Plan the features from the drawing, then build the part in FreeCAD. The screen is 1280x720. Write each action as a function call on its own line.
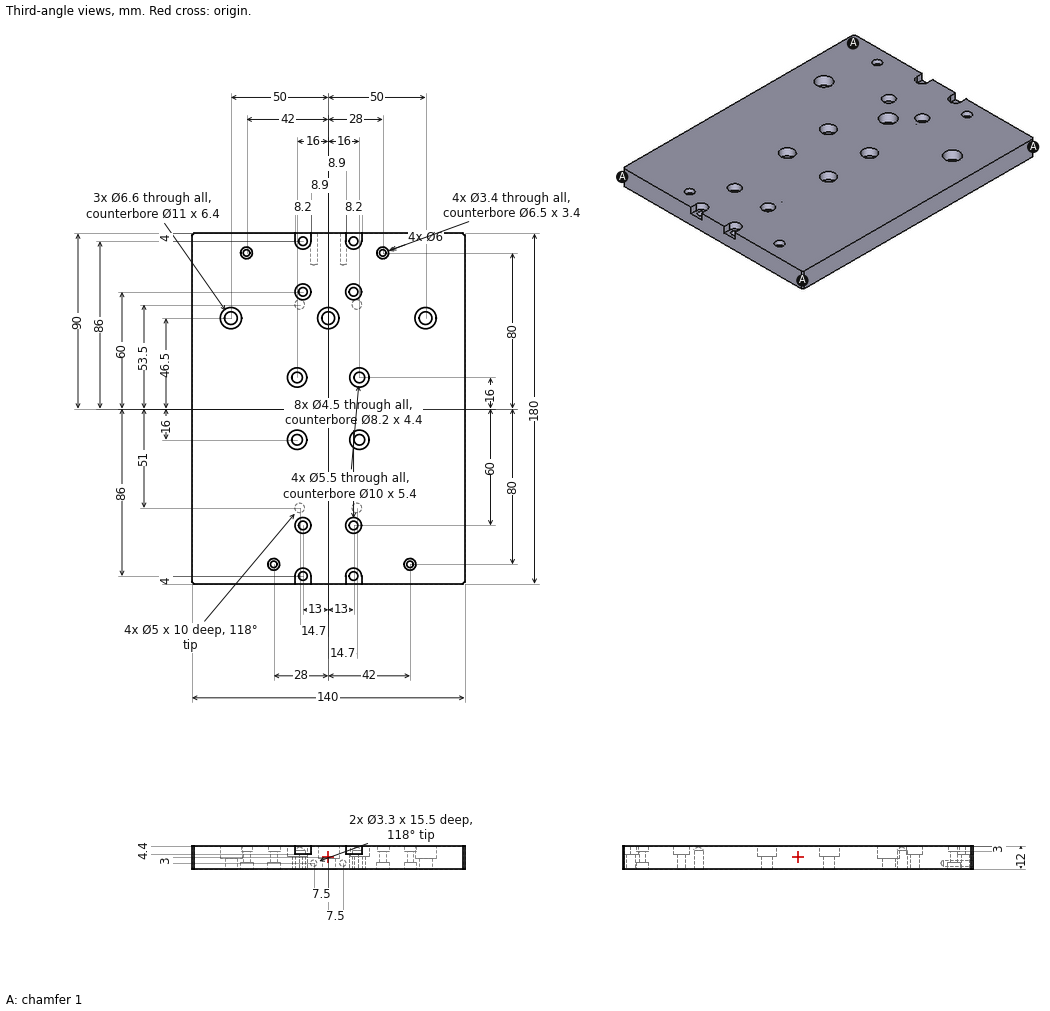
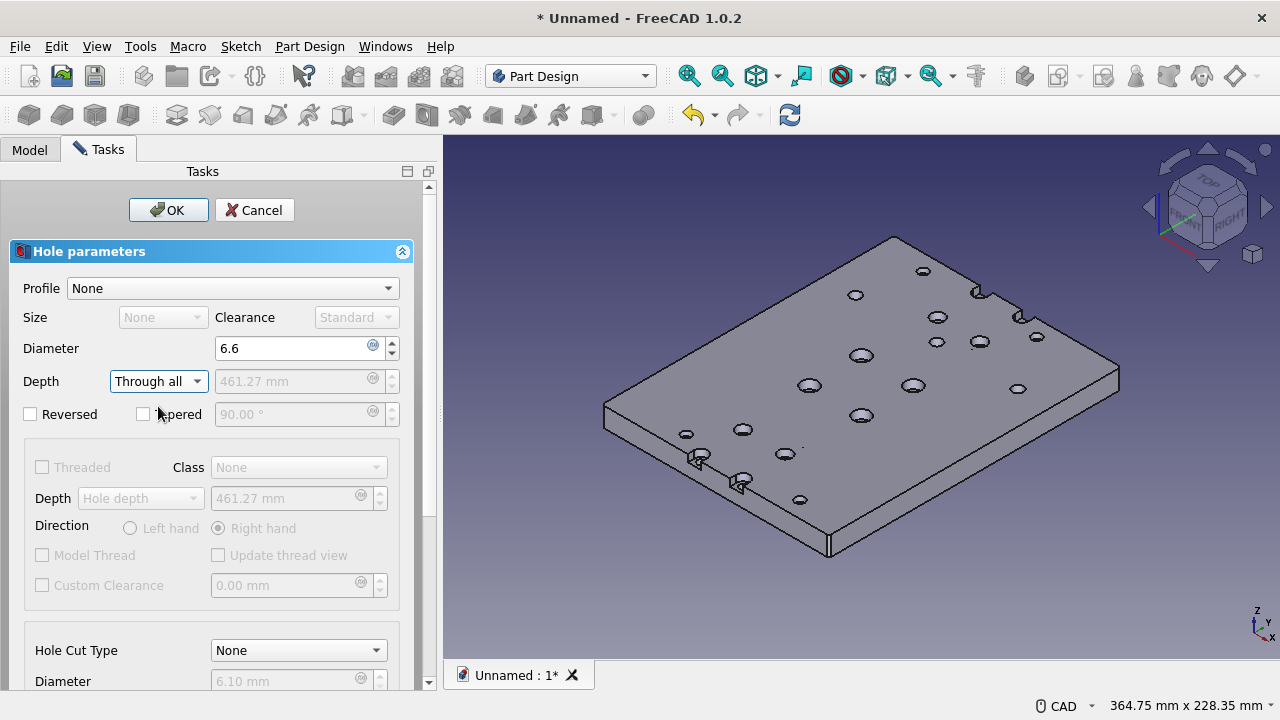
click(300, 650)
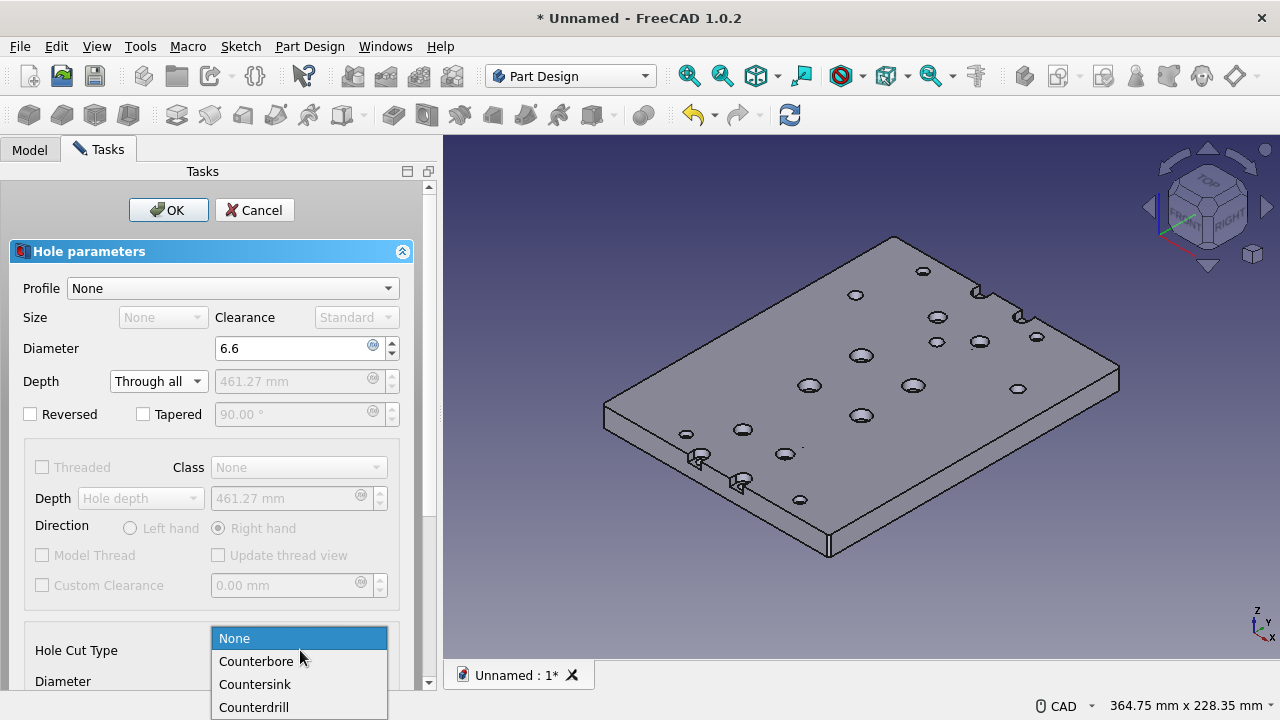
click(298, 662)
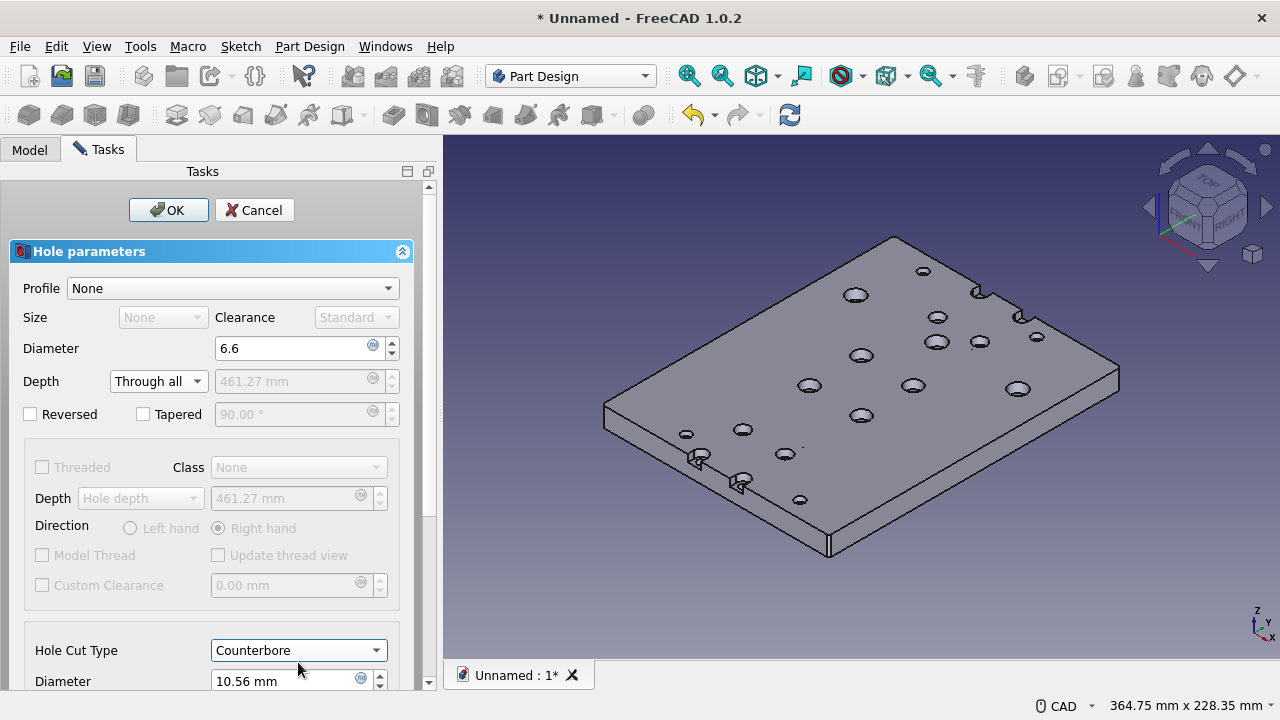
scroll(429, 436, down, 2)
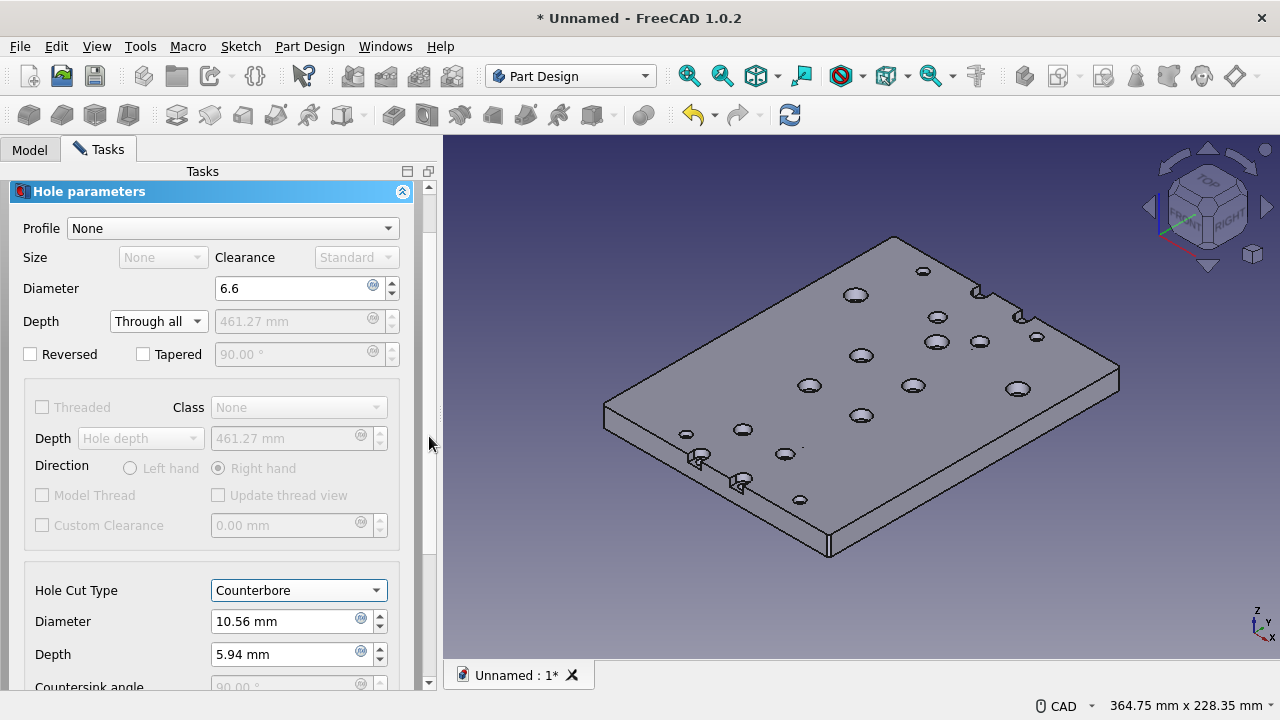
triple_click(292, 562)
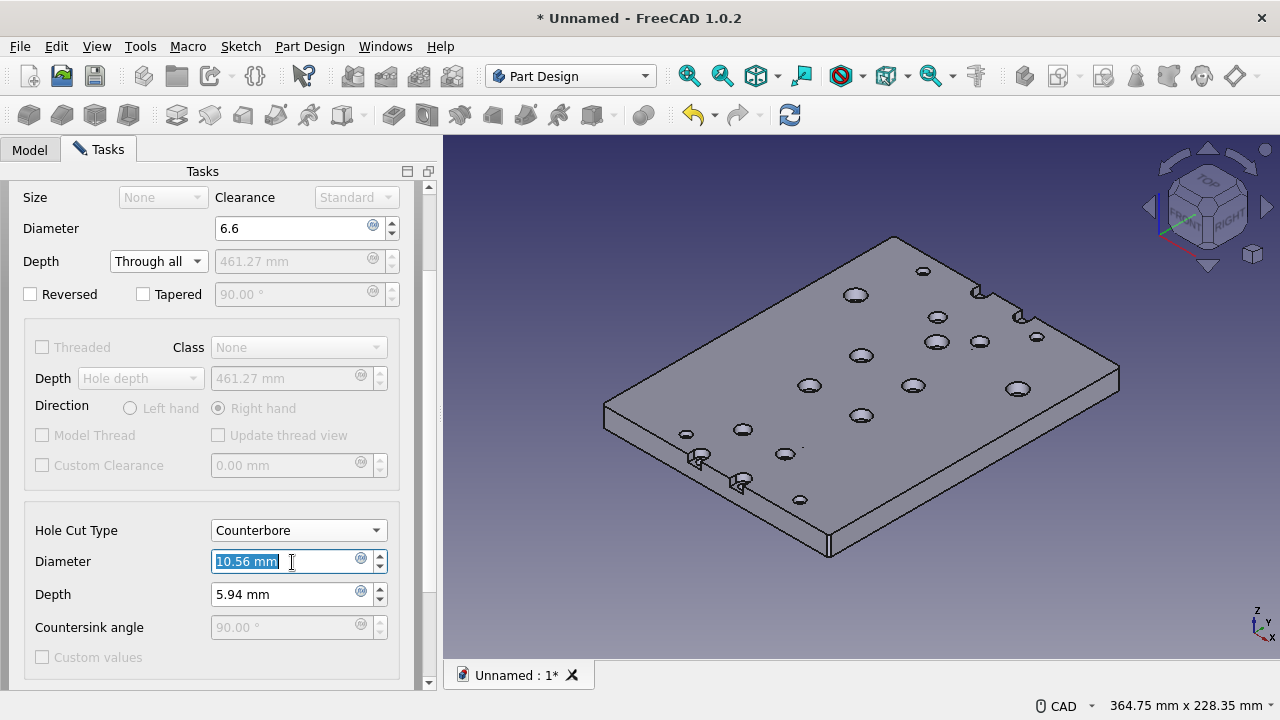
text(11)
key(Tab)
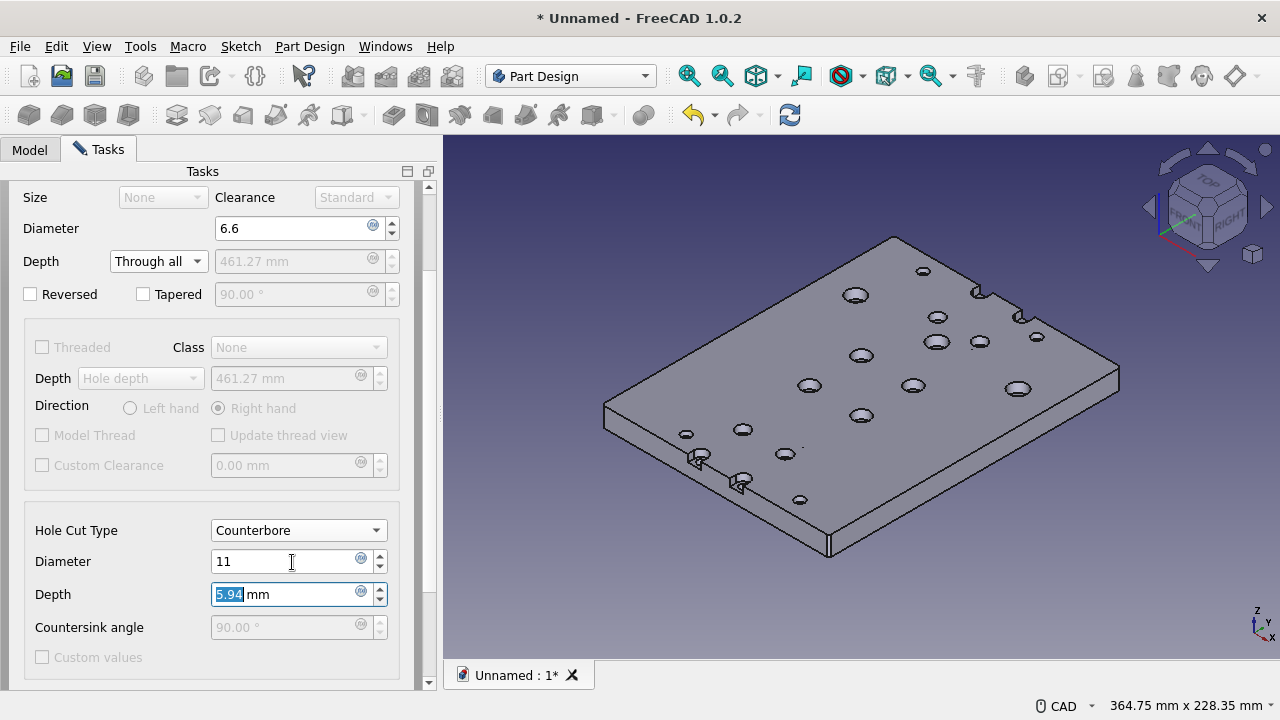
text(6.4)
key(Tab)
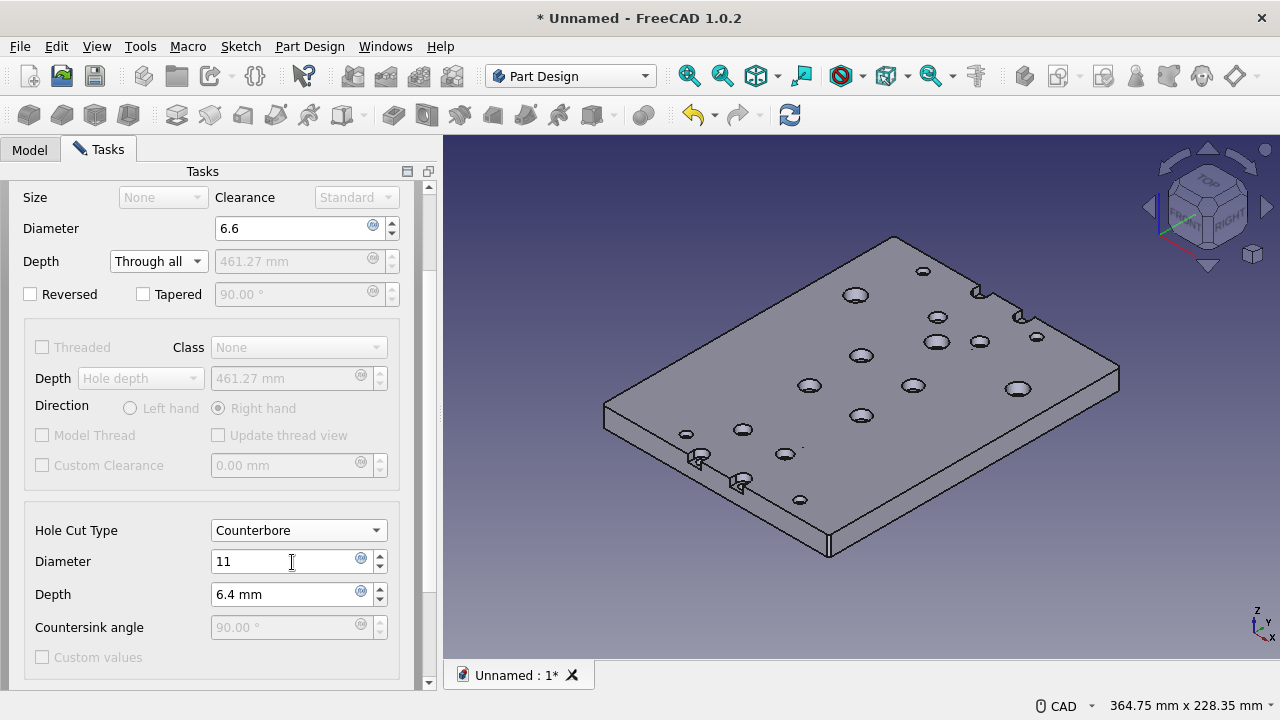
scroll(429, 436, up, 3)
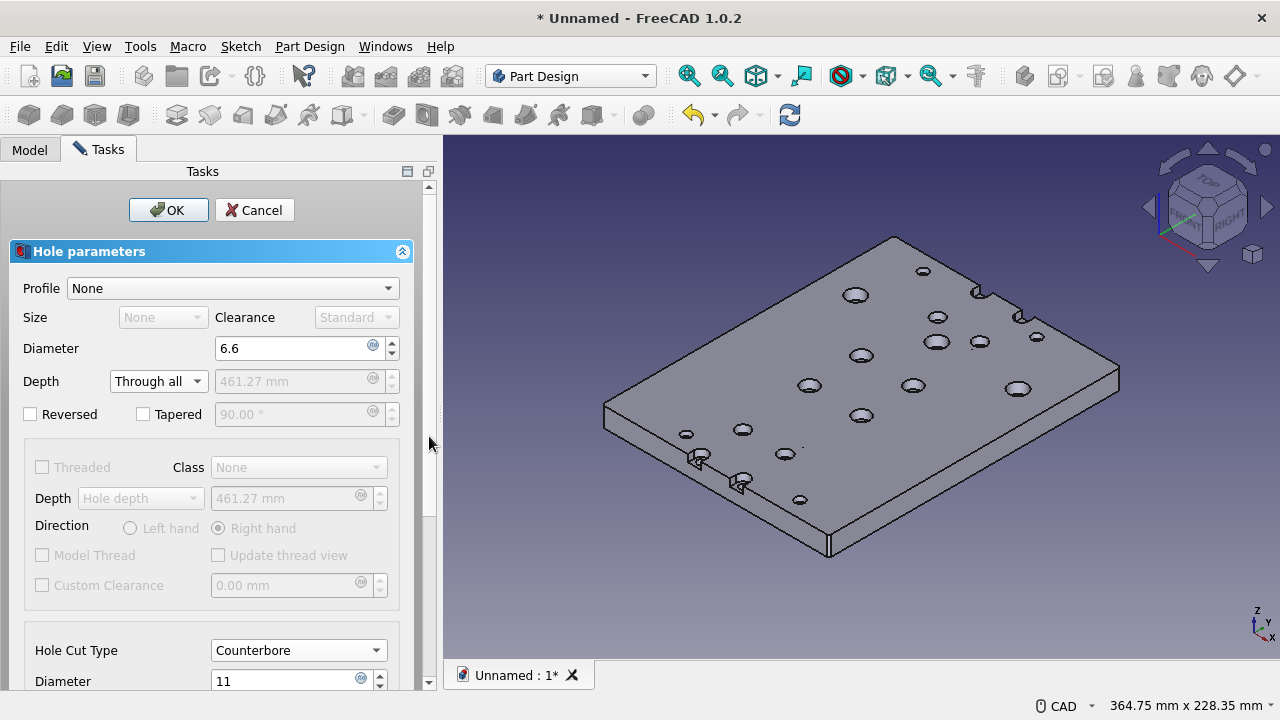
click(169, 210)